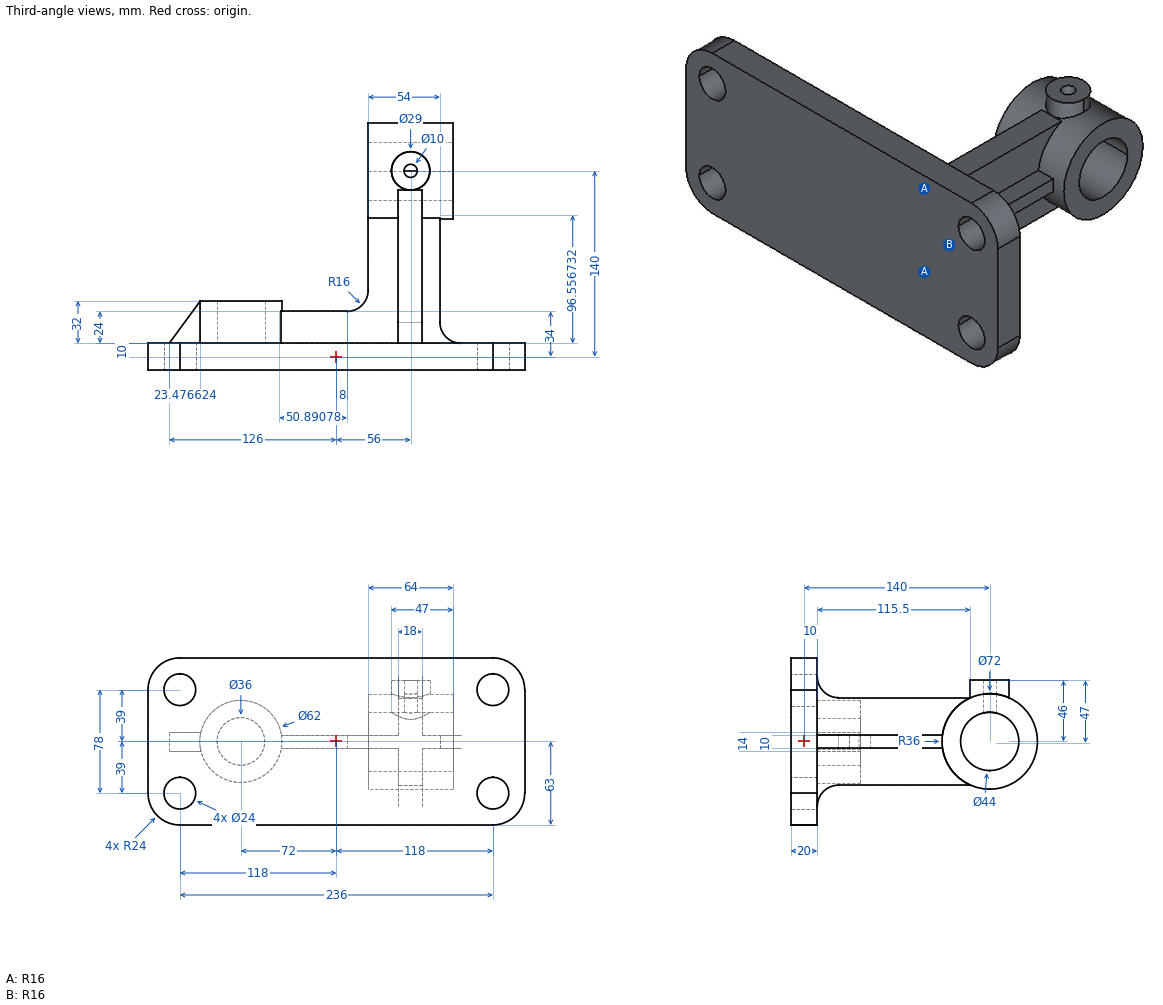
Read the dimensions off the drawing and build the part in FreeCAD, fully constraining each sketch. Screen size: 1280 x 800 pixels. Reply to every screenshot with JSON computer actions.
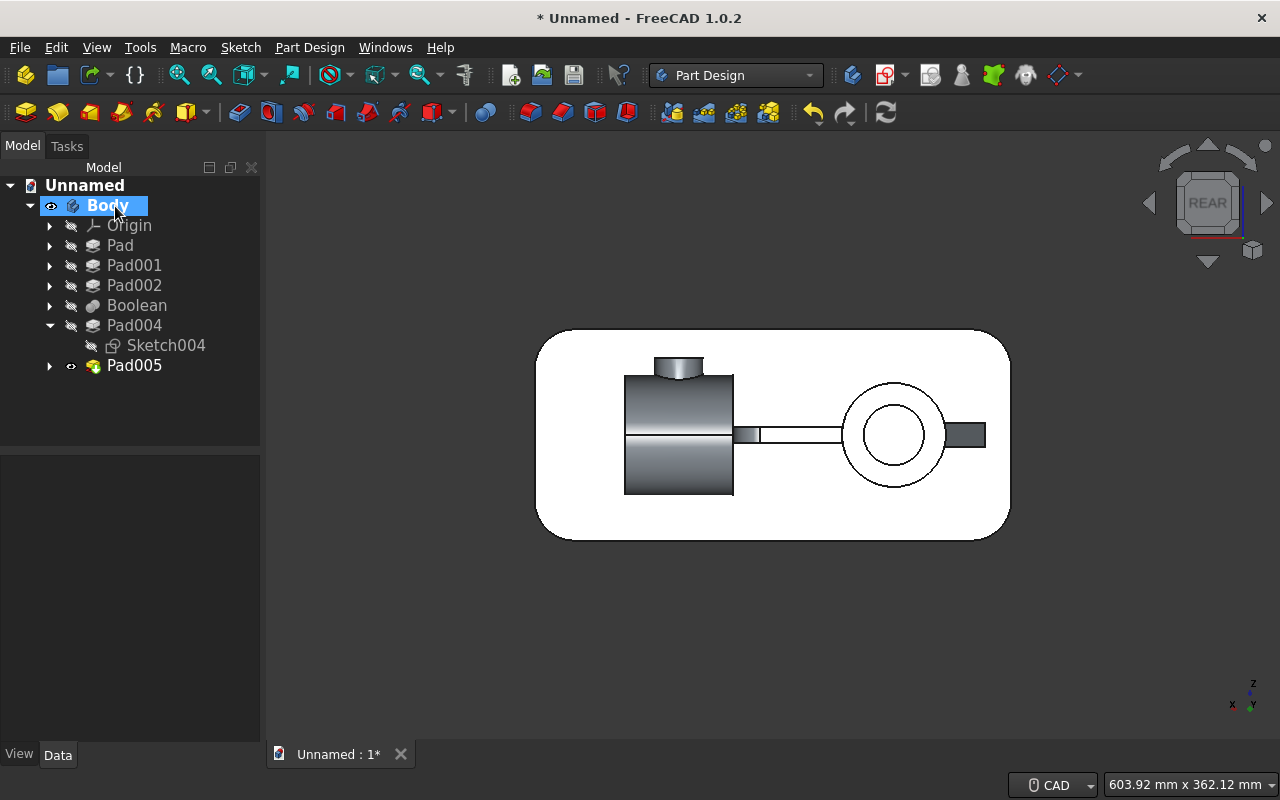
{"action": "left_click", "coordinate": [50, 226]}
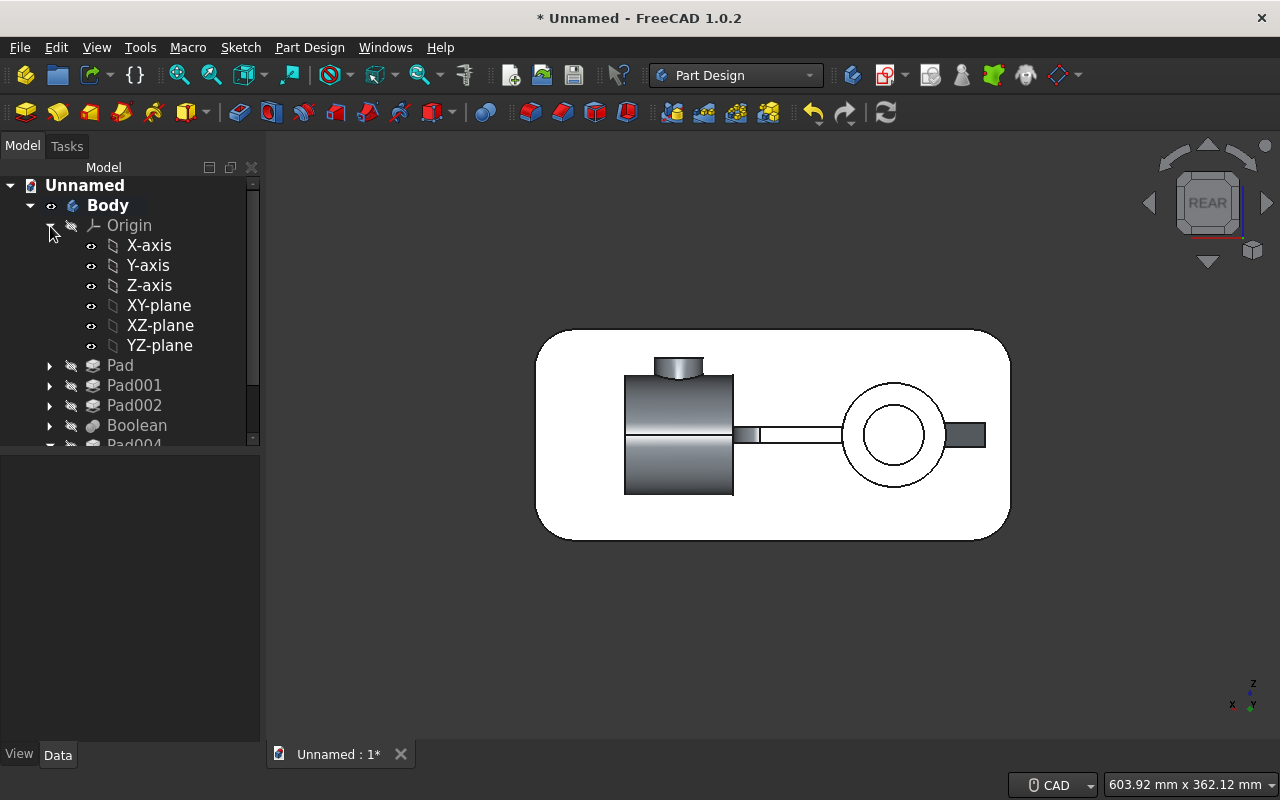
{"action": "left_click", "coordinate": [136, 346]}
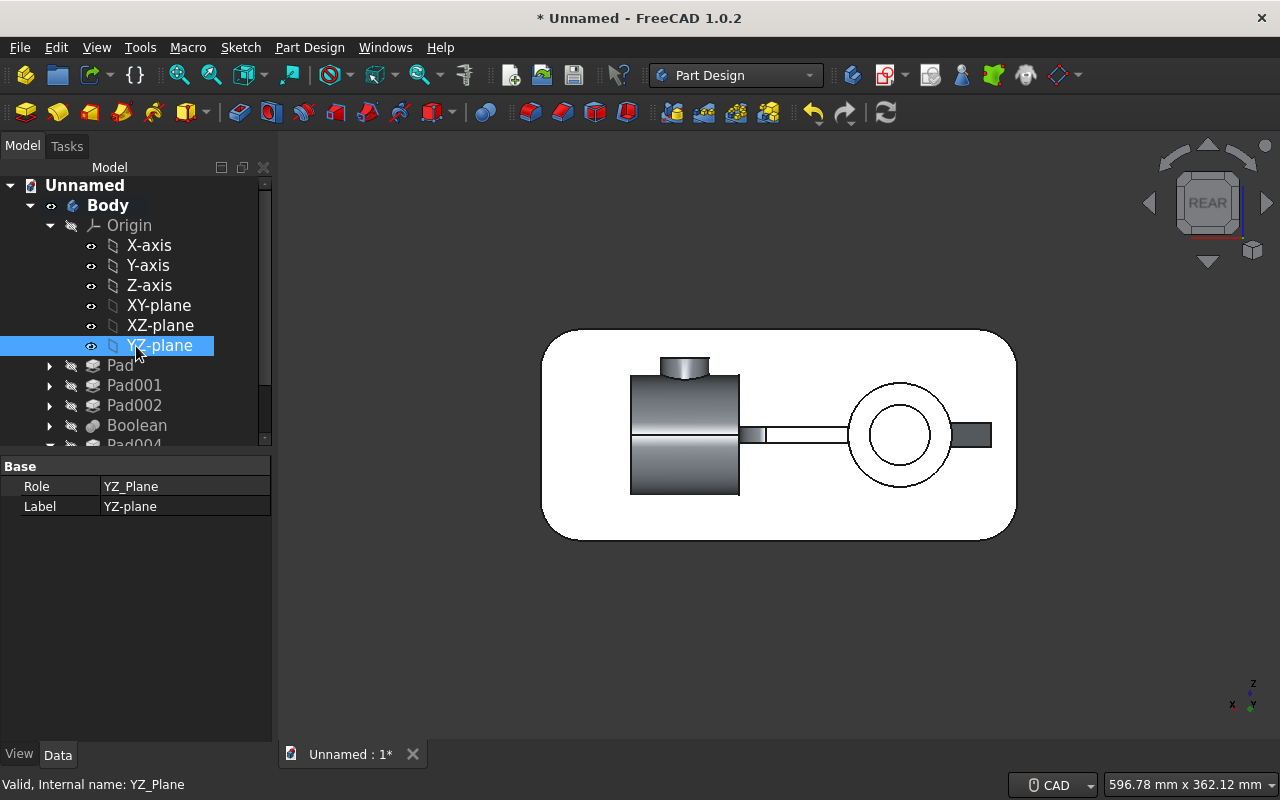
{"action": "left_click", "coordinate": [1058, 76]}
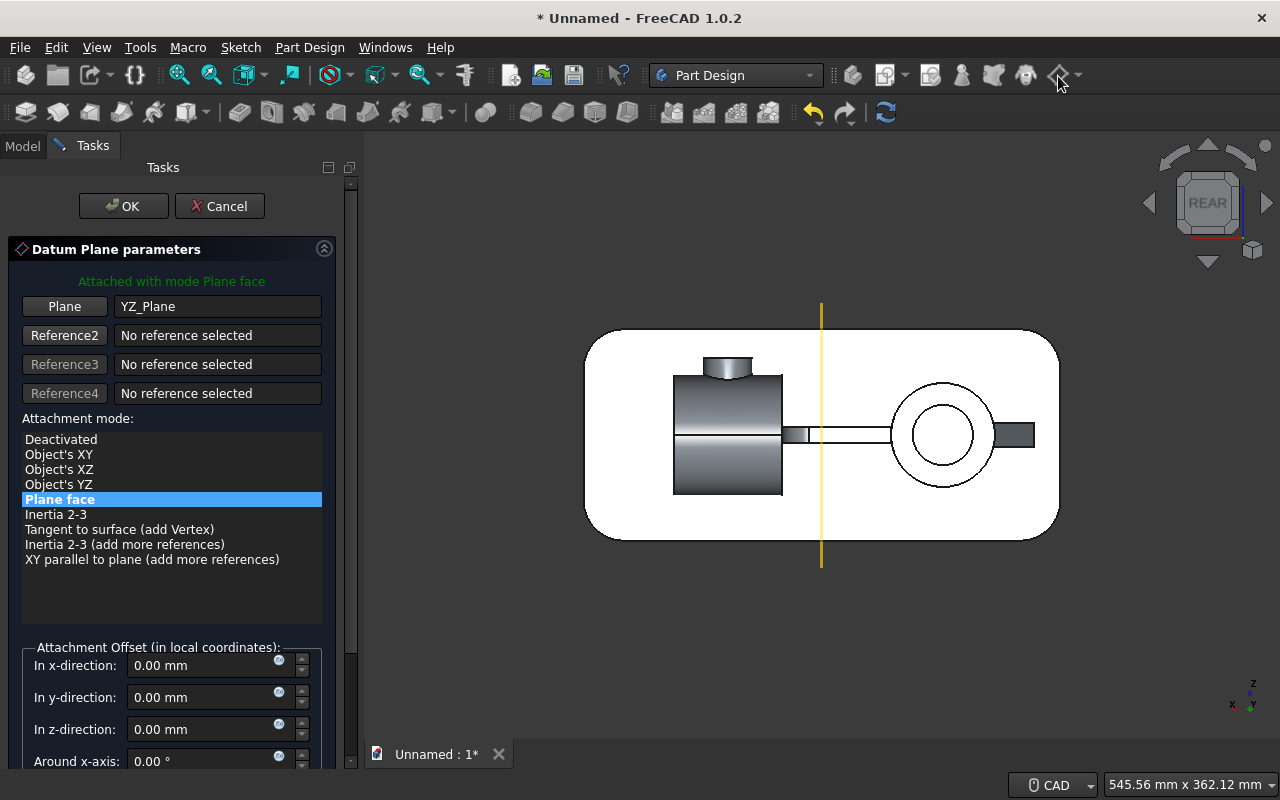
{"action": "triple_click", "coordinate": [210, 729]}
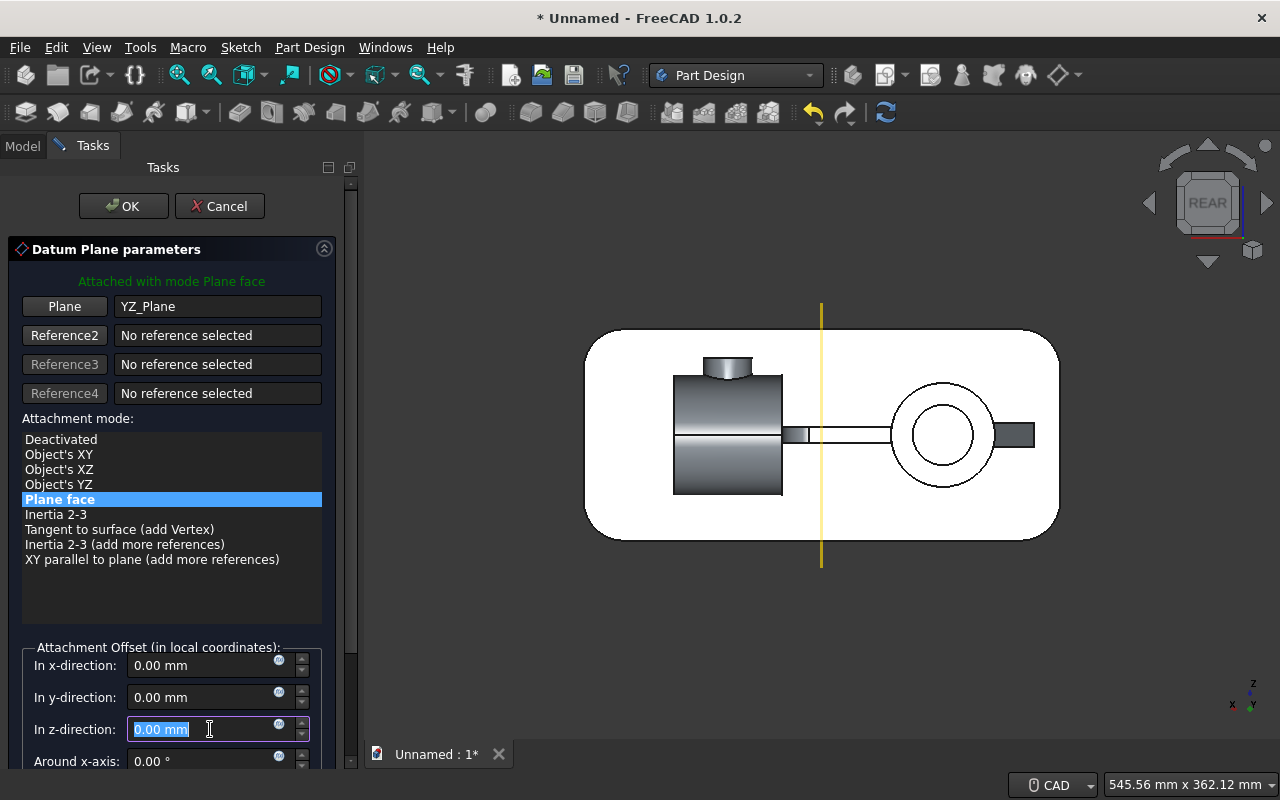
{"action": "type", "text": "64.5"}
{"action": "key", "text": "Tab"}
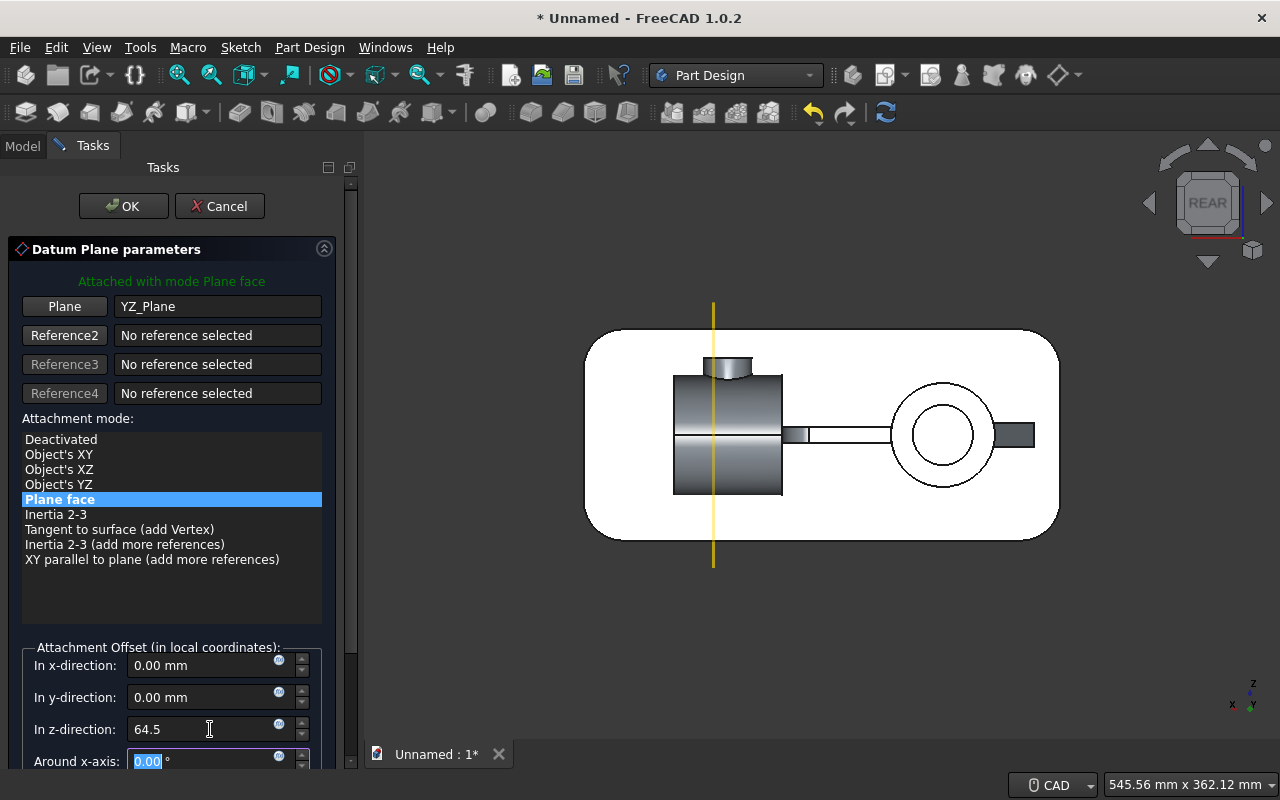
{"action": "left_click", "coordinate": [124, 206]}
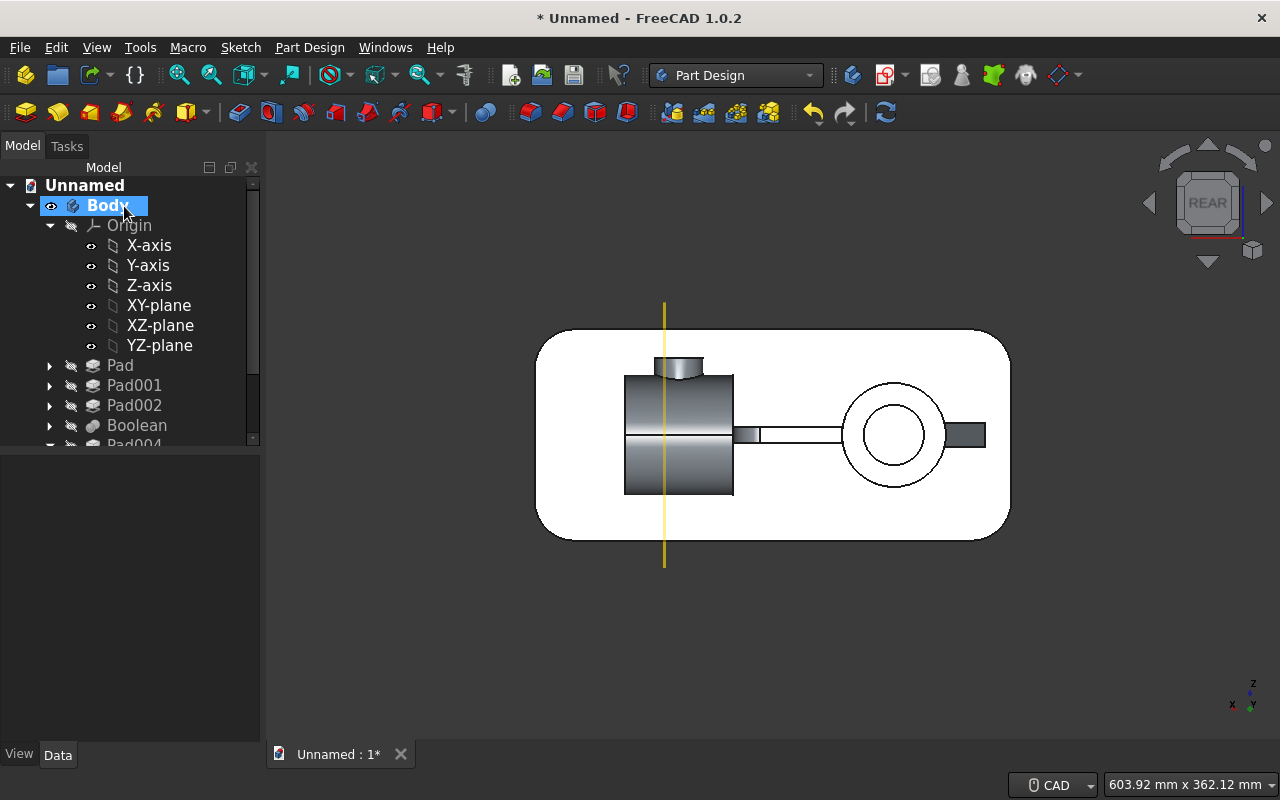
{"action": "scroll", "coordinate": [100, 321], "scroll_direction": "down", "scroll_amount": 3}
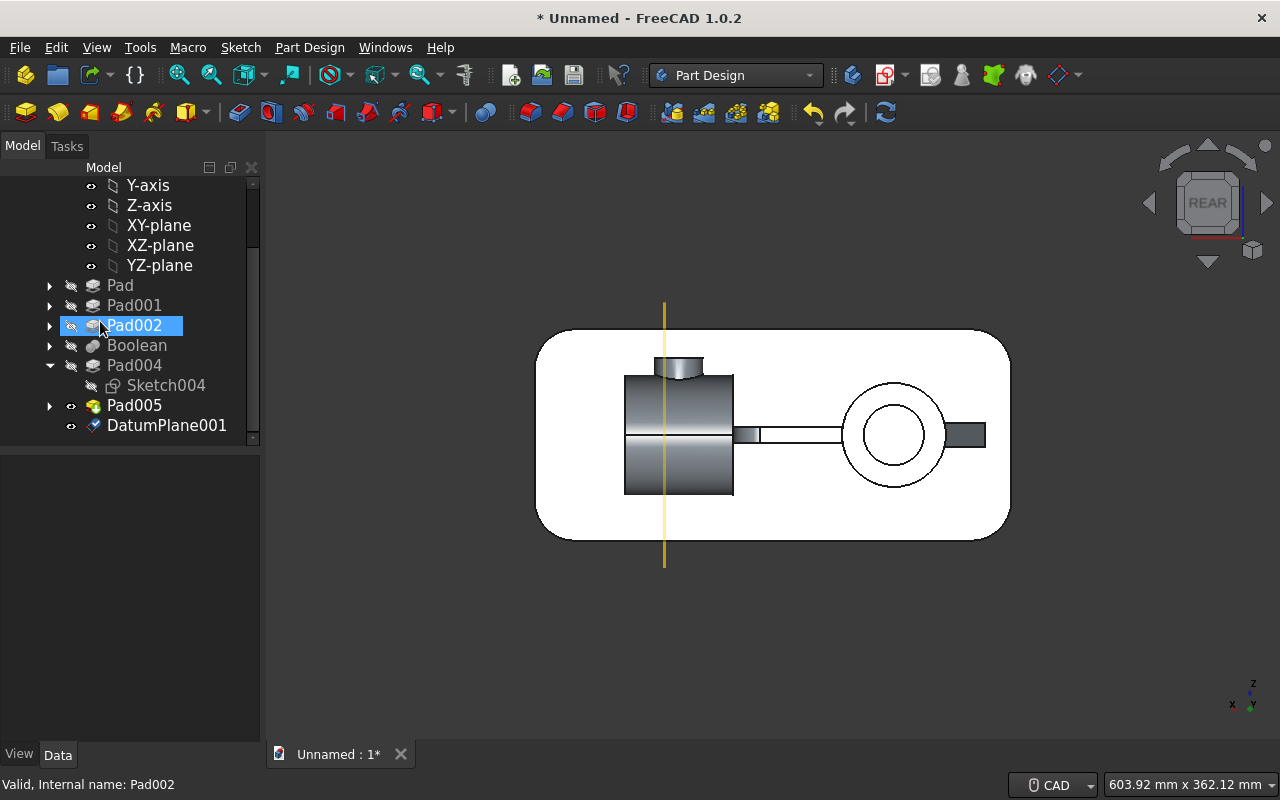
{"action": "left_click", "coordinate": [116, 426]}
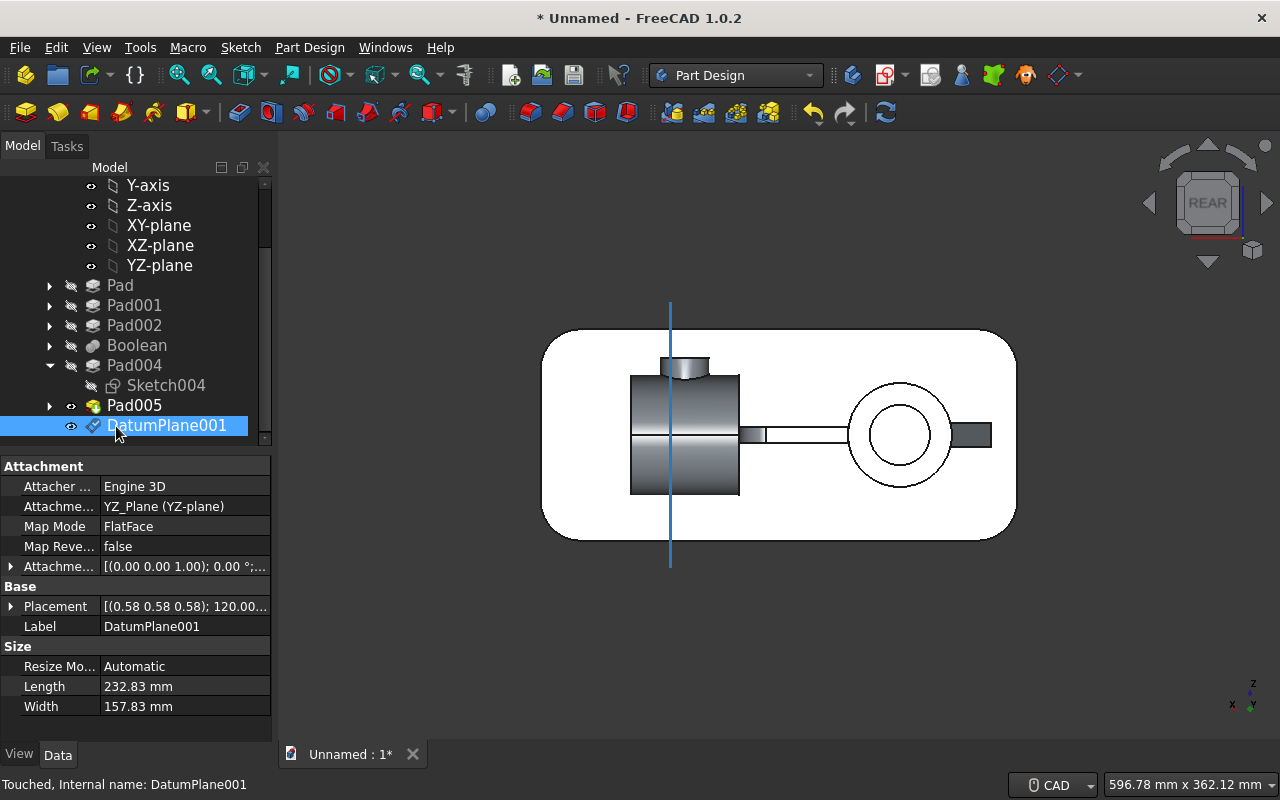
{"action": "left_click", "coordinate": [886, 76]}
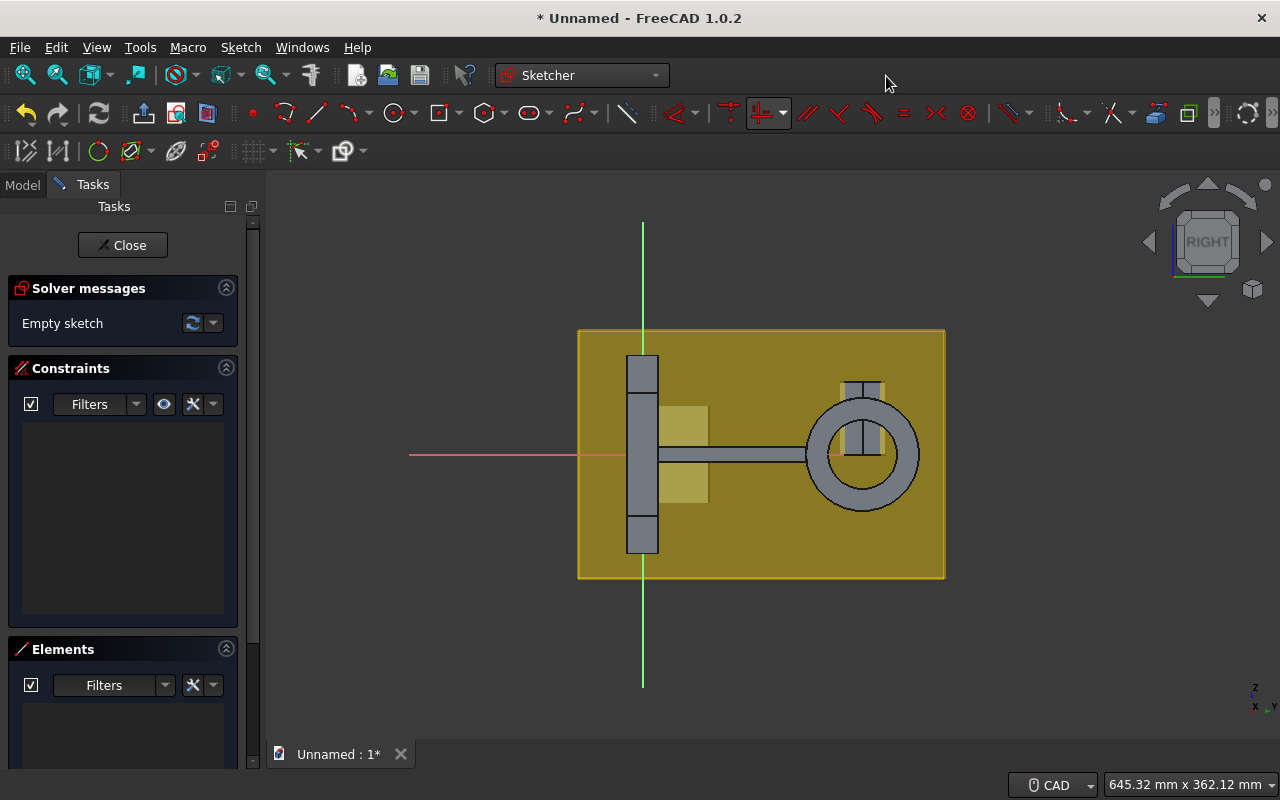
{"action": "left_click", "coordinate": [208, 114]}